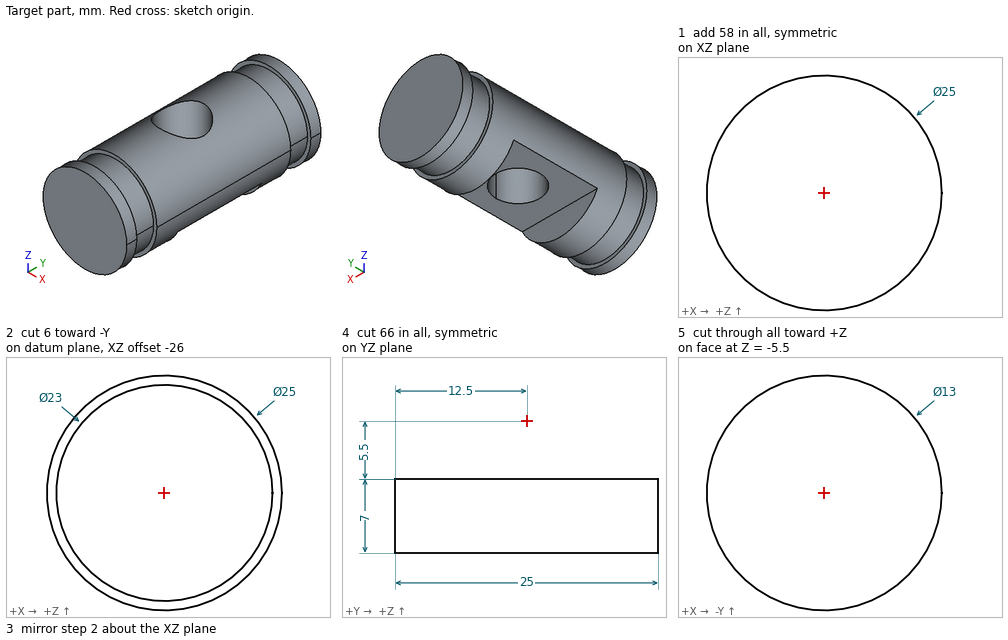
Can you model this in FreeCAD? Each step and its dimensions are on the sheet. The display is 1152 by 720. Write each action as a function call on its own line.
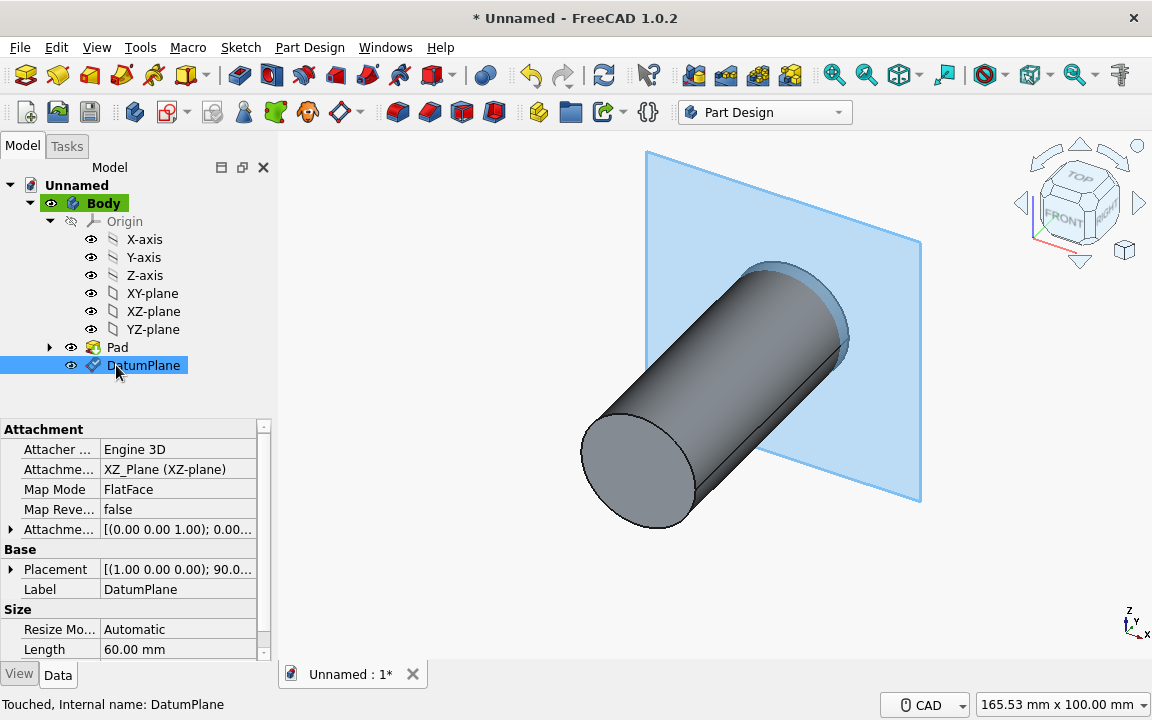
click(168, 112)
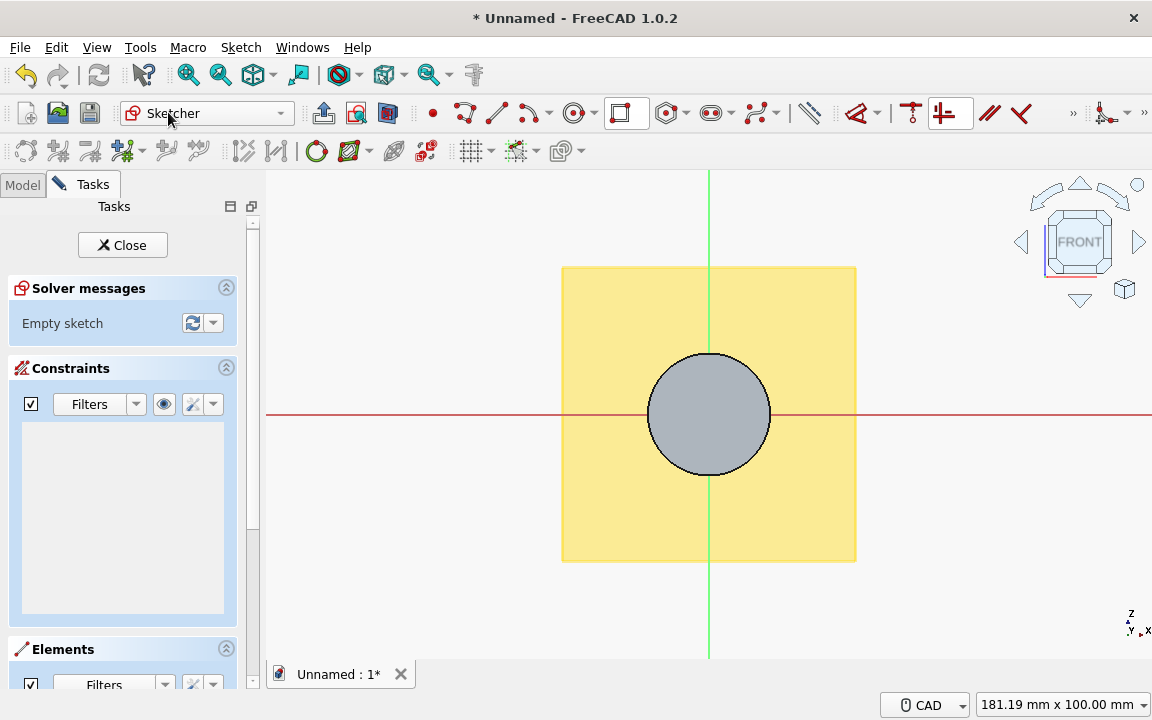
click(388, 114)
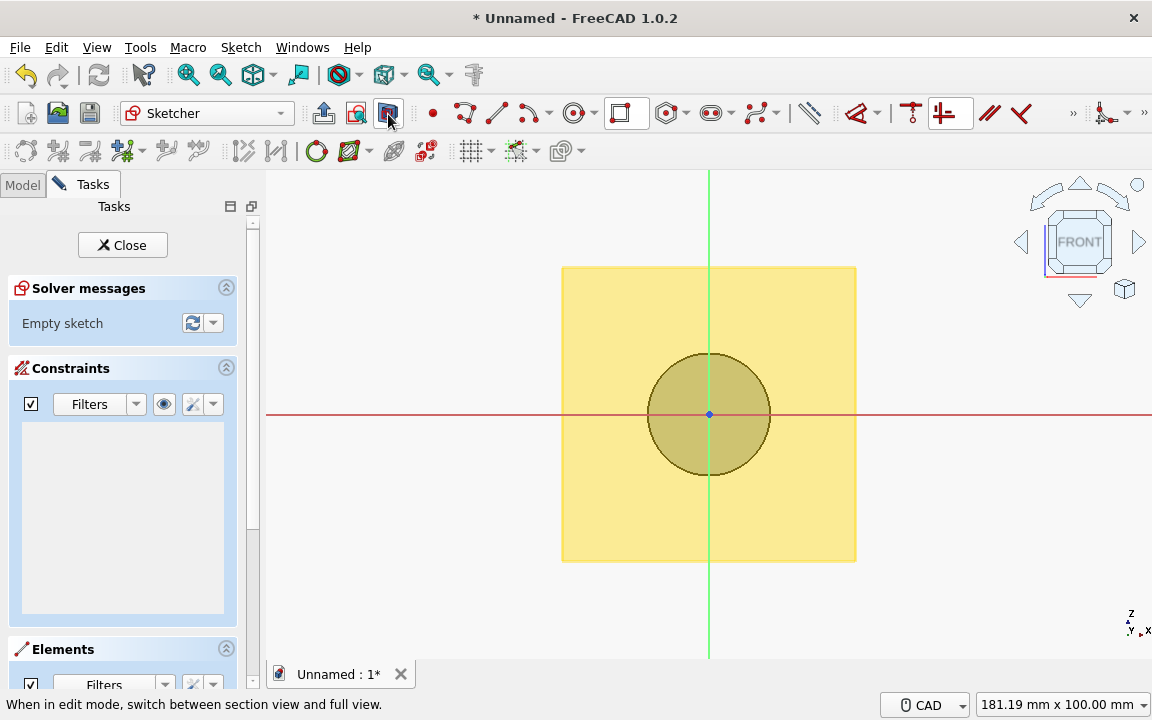
scroll(749, 415, up, 5)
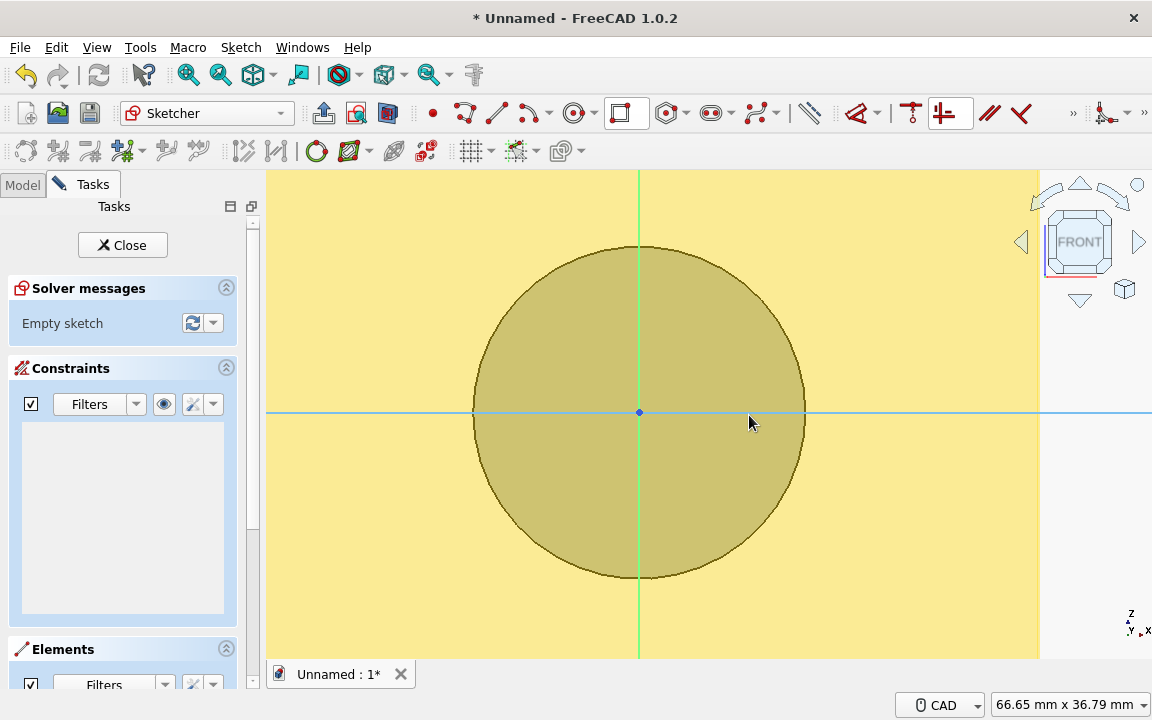
click(574, 114)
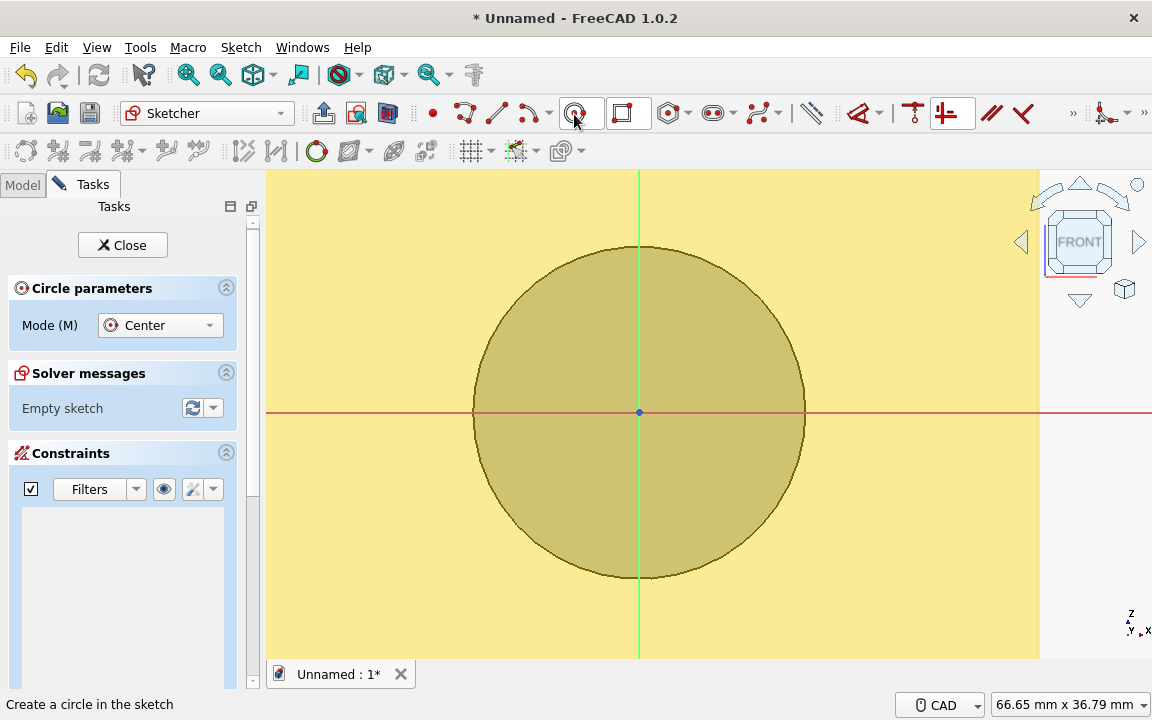
click(639, 413)
click(757, 295)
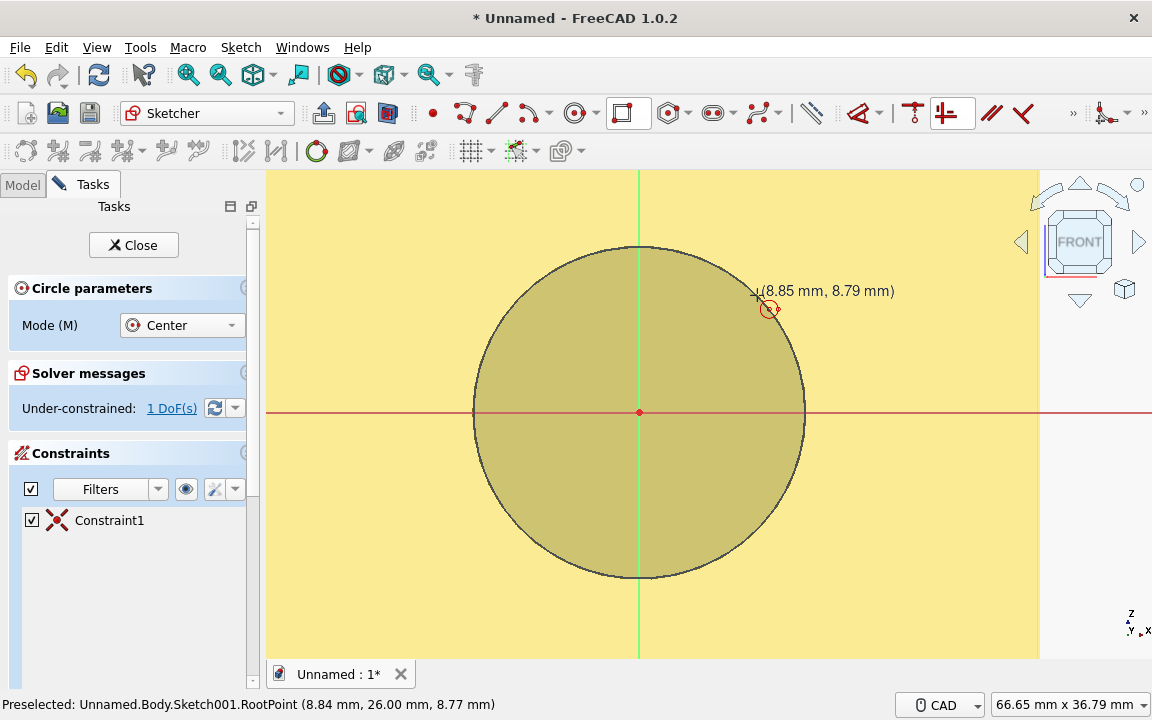
click(639, 413)
click(692, 269)
key(Escape)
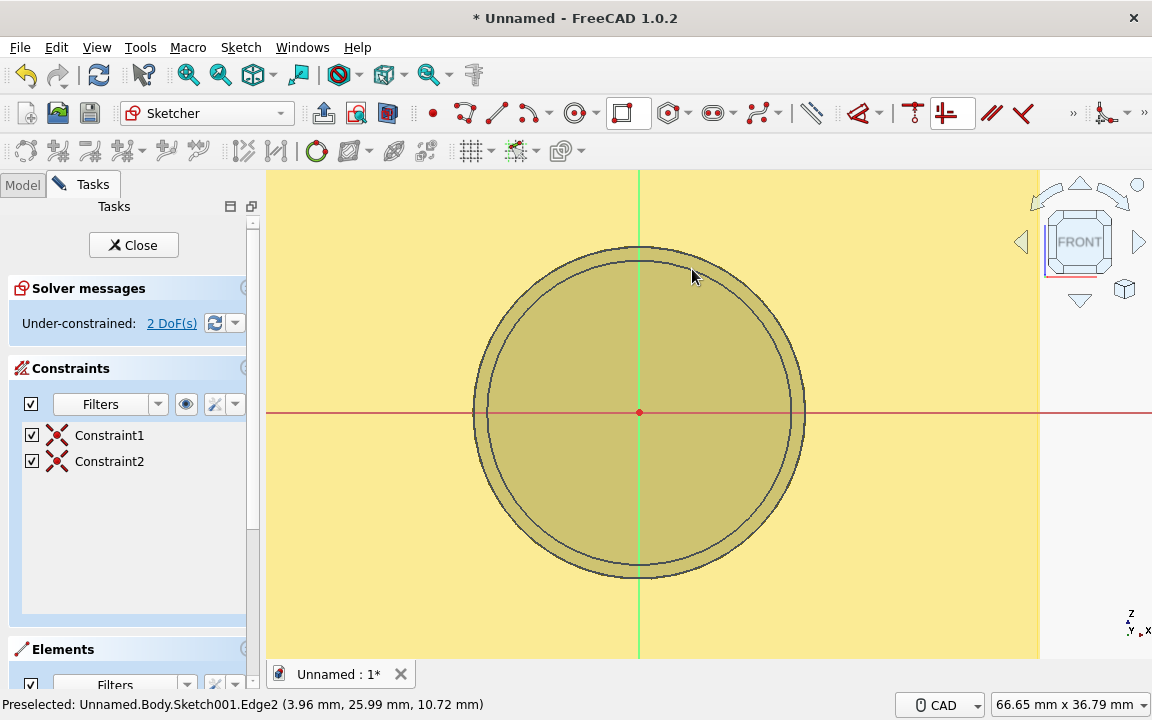
click(858, 114)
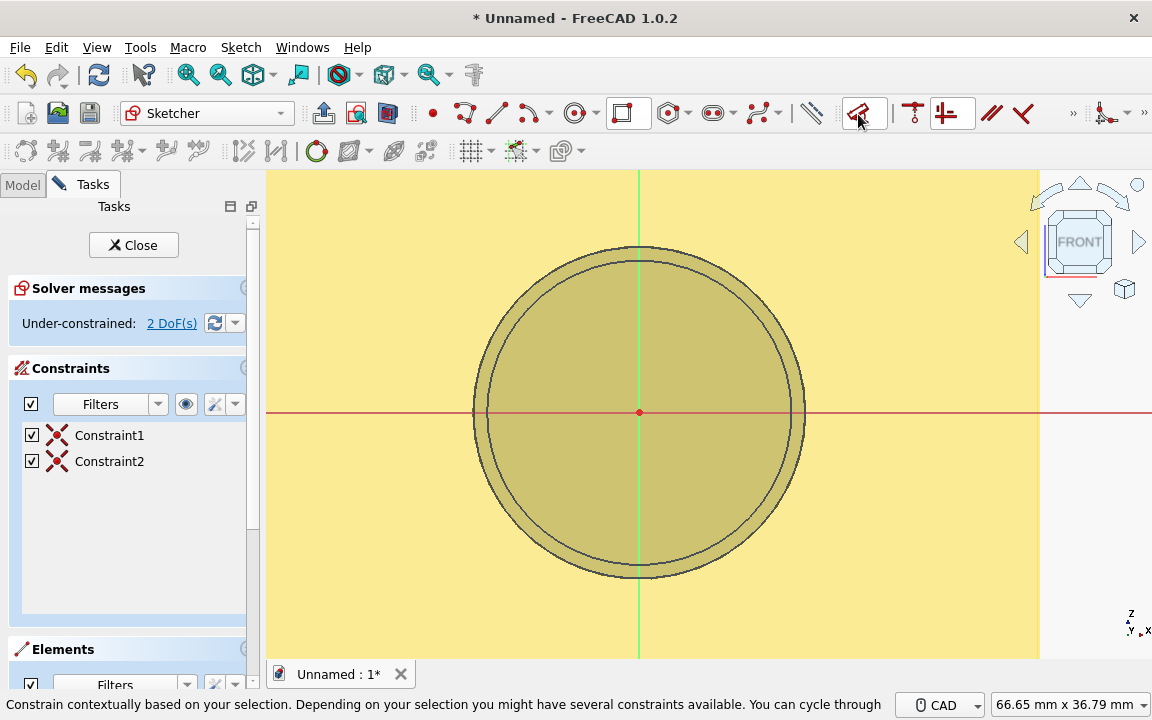
click(756, 295)
click(779, 272)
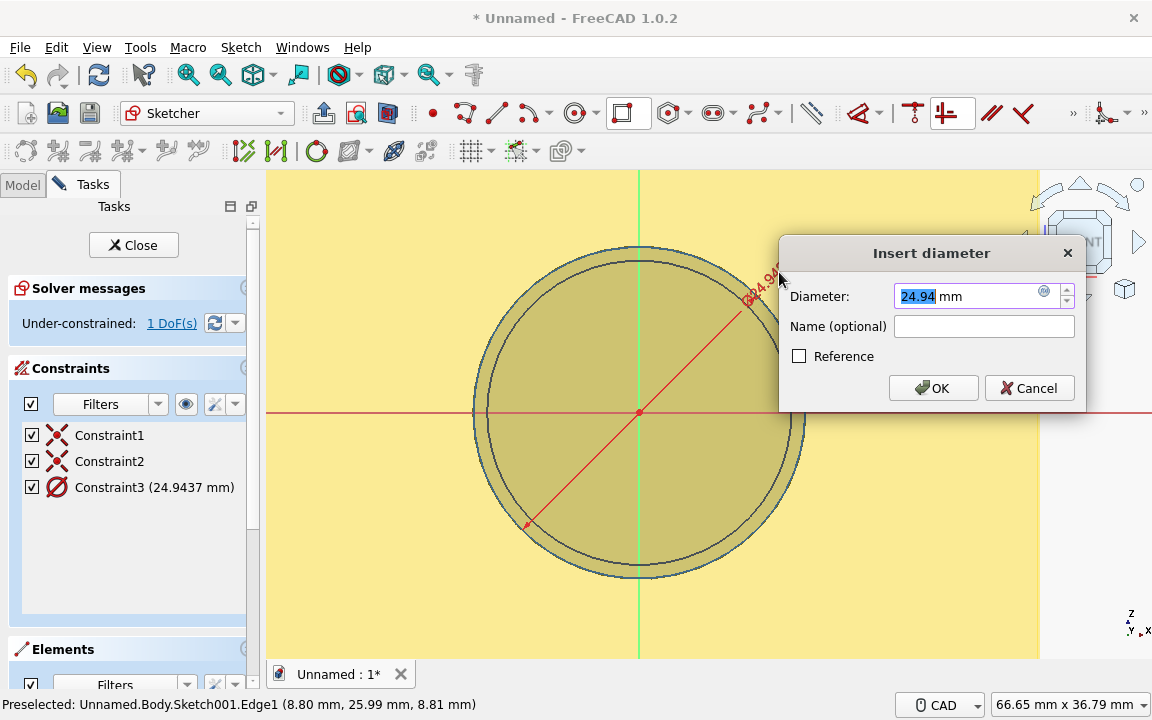
text(25)
key(Return)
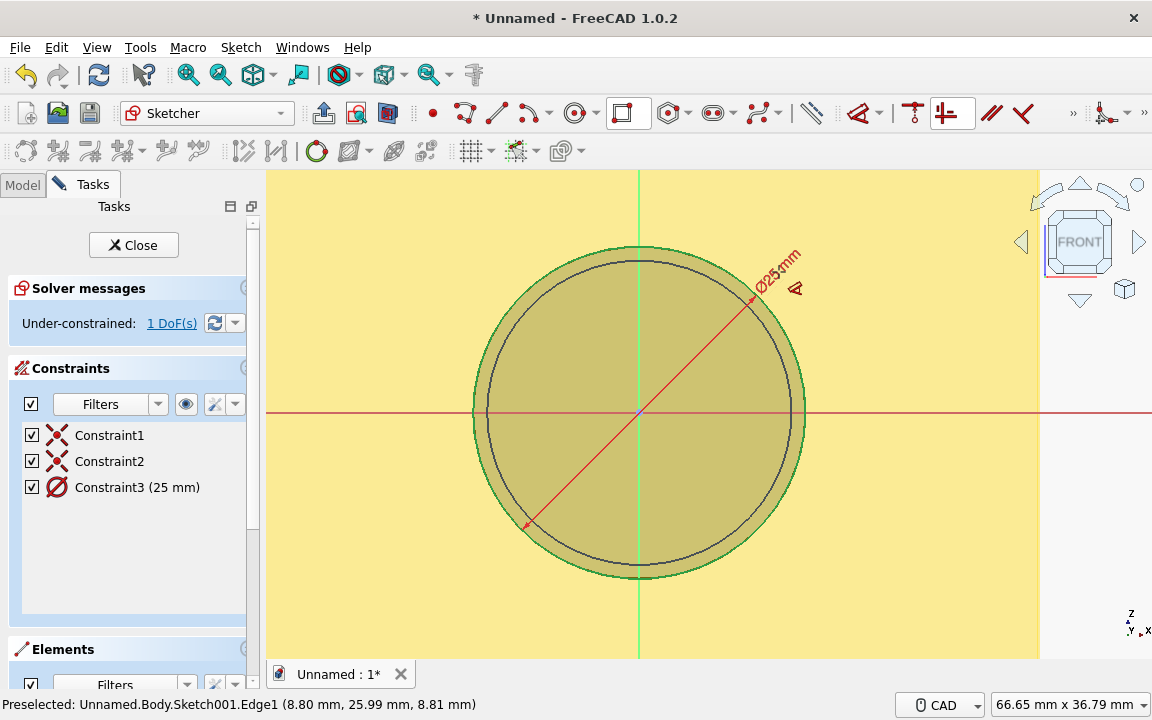
click(747, 305)
click(816, 361)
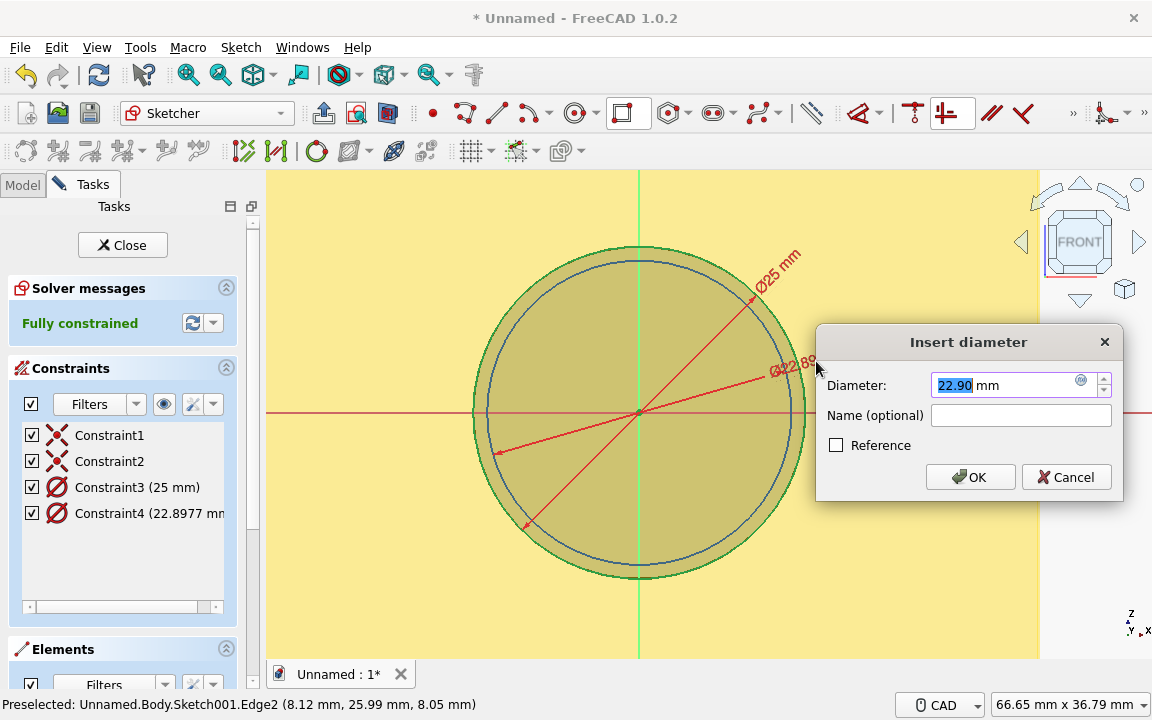
text(23)
key(Return)
key(Escape)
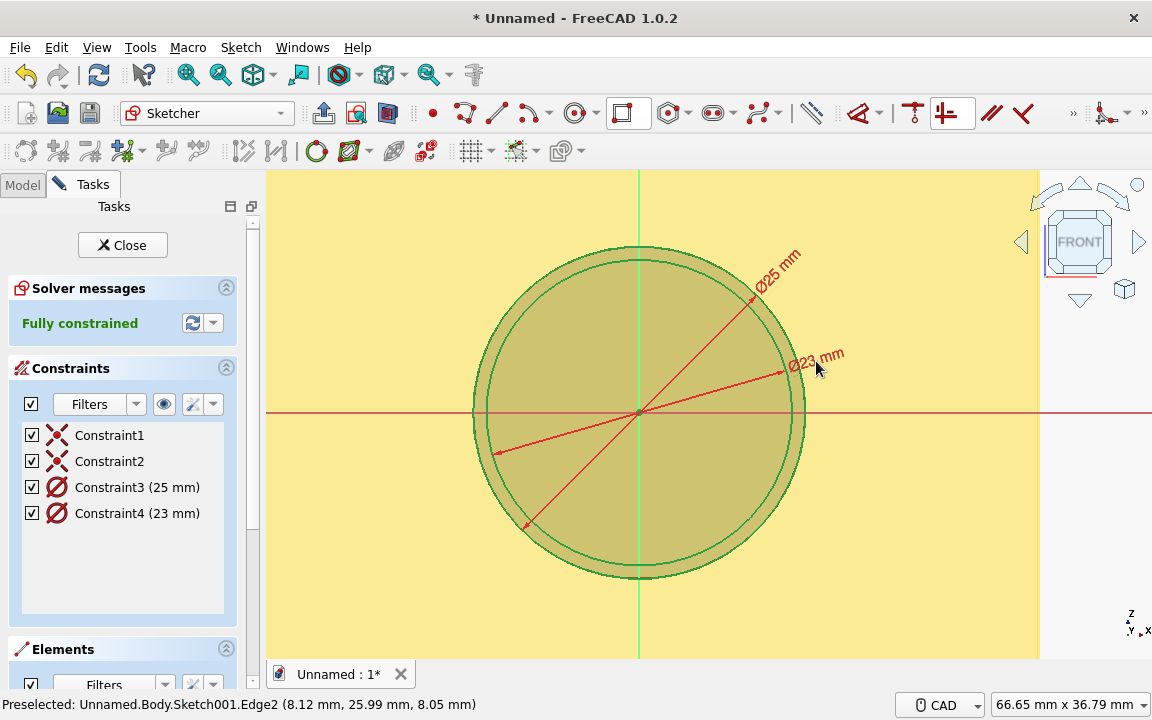
click(123, 245)